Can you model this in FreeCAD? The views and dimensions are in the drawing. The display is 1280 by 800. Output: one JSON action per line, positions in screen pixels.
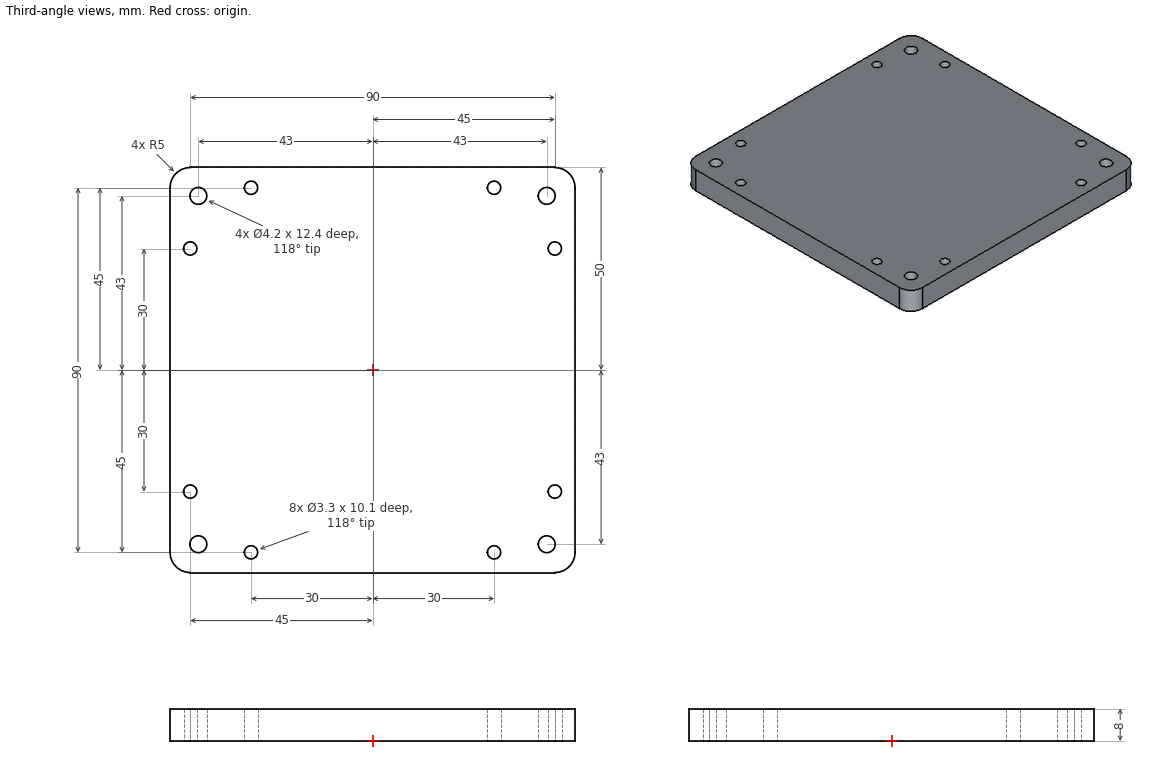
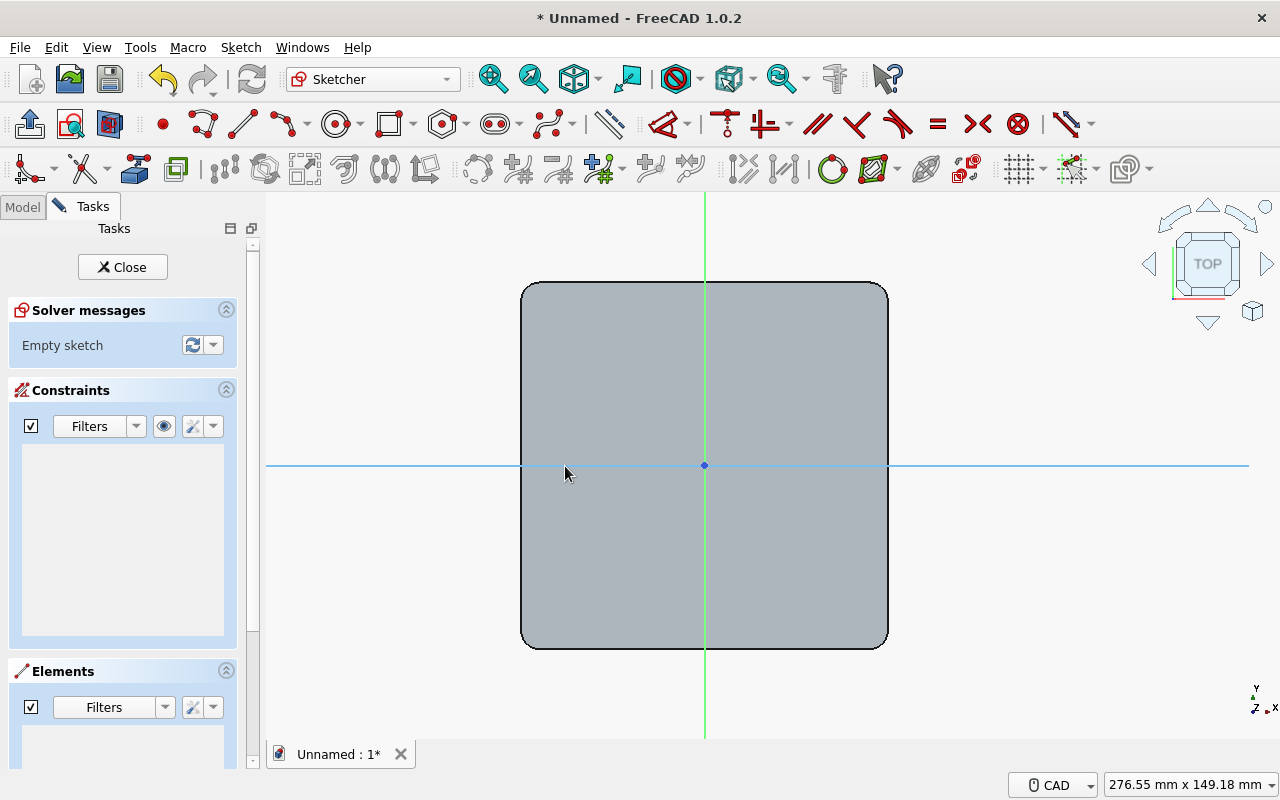
{"action": "key", "text": "g c"}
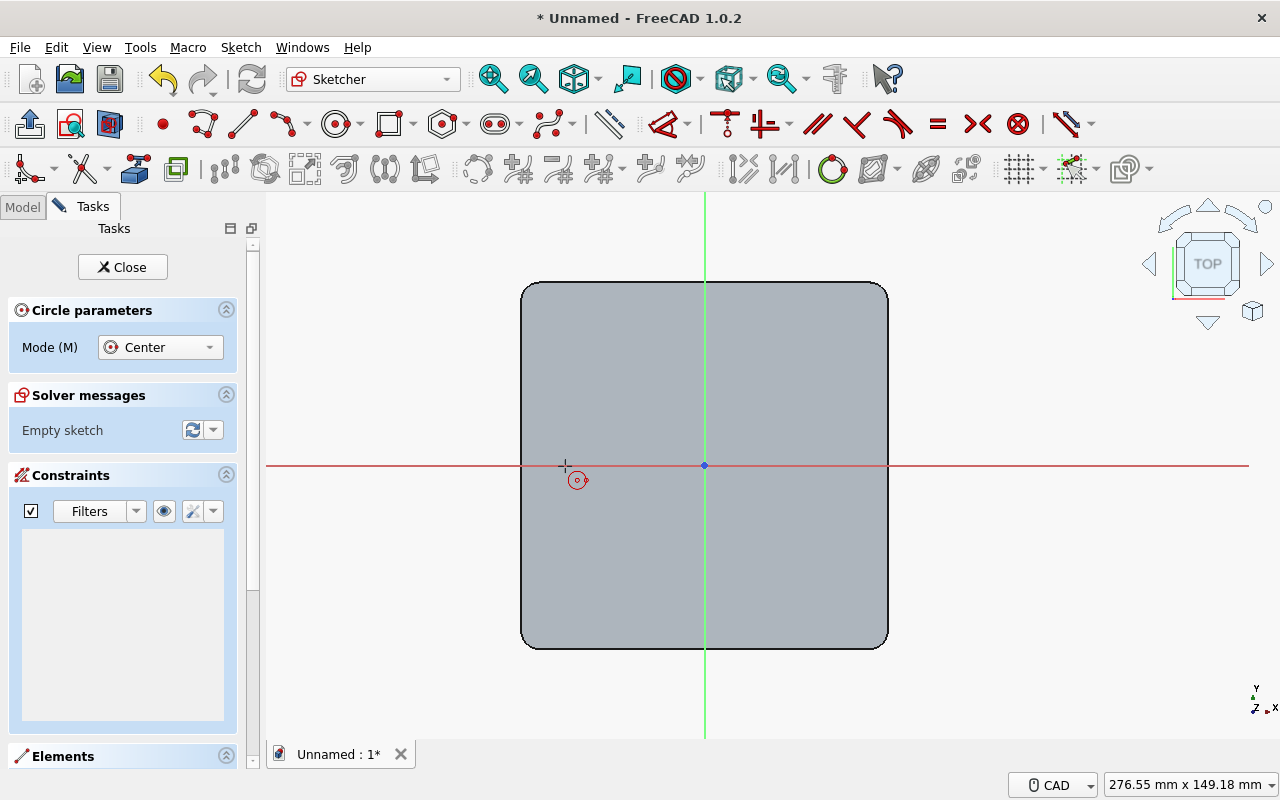
{"action": "scroll", "coordinate": [547, 308], "scroll_direction": "up", "scroll_amount": 6}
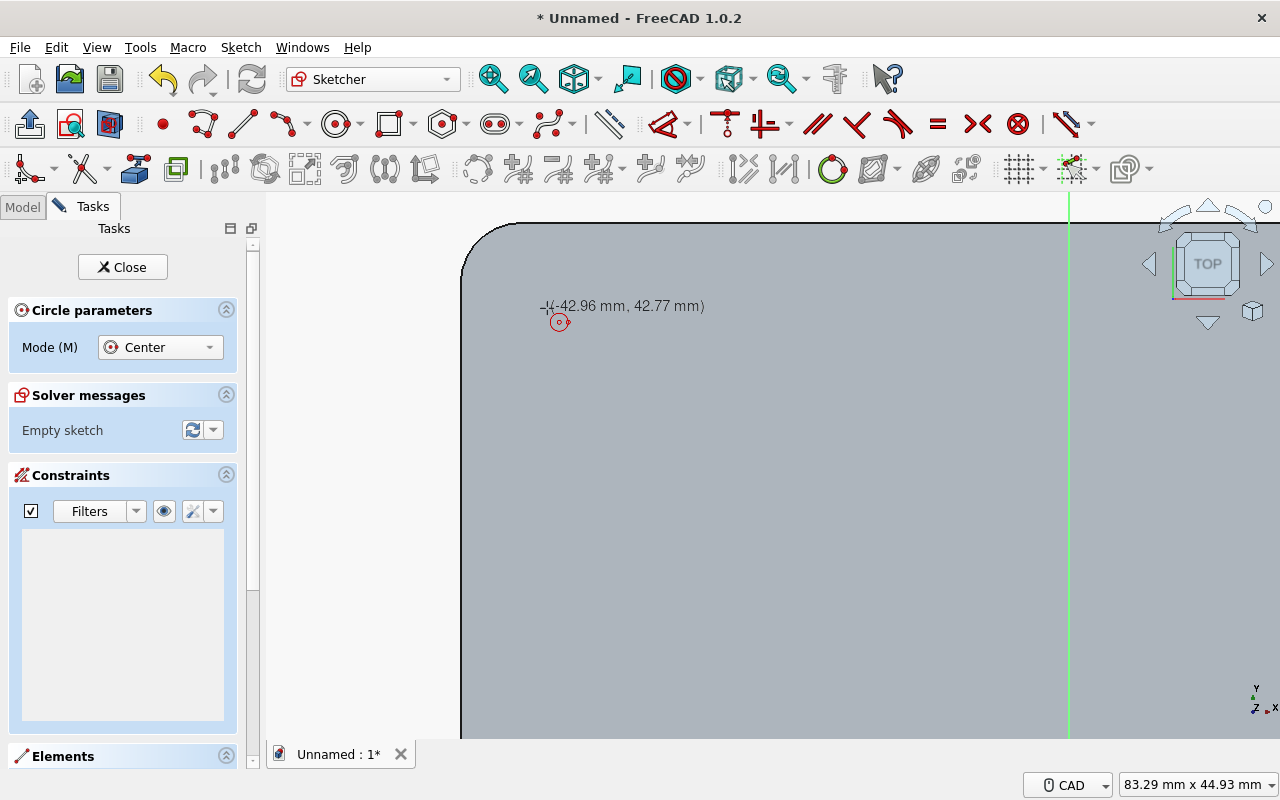
{"action": "left_click", "coordinate": [546, 308]}
{"action": "mouse_move", "coordinate": [564, 290]}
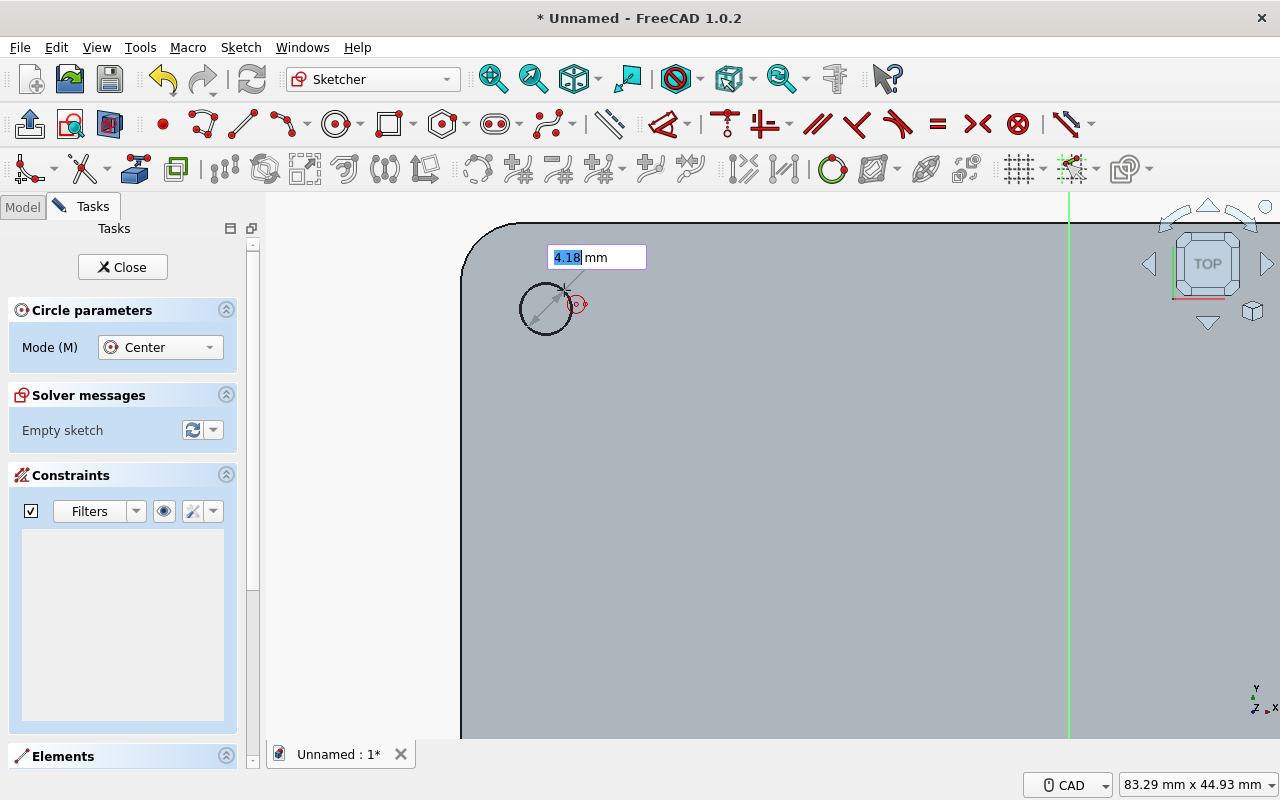
{"action": "type", "text": "4.2"}
{"action": "key", "text": "Return"}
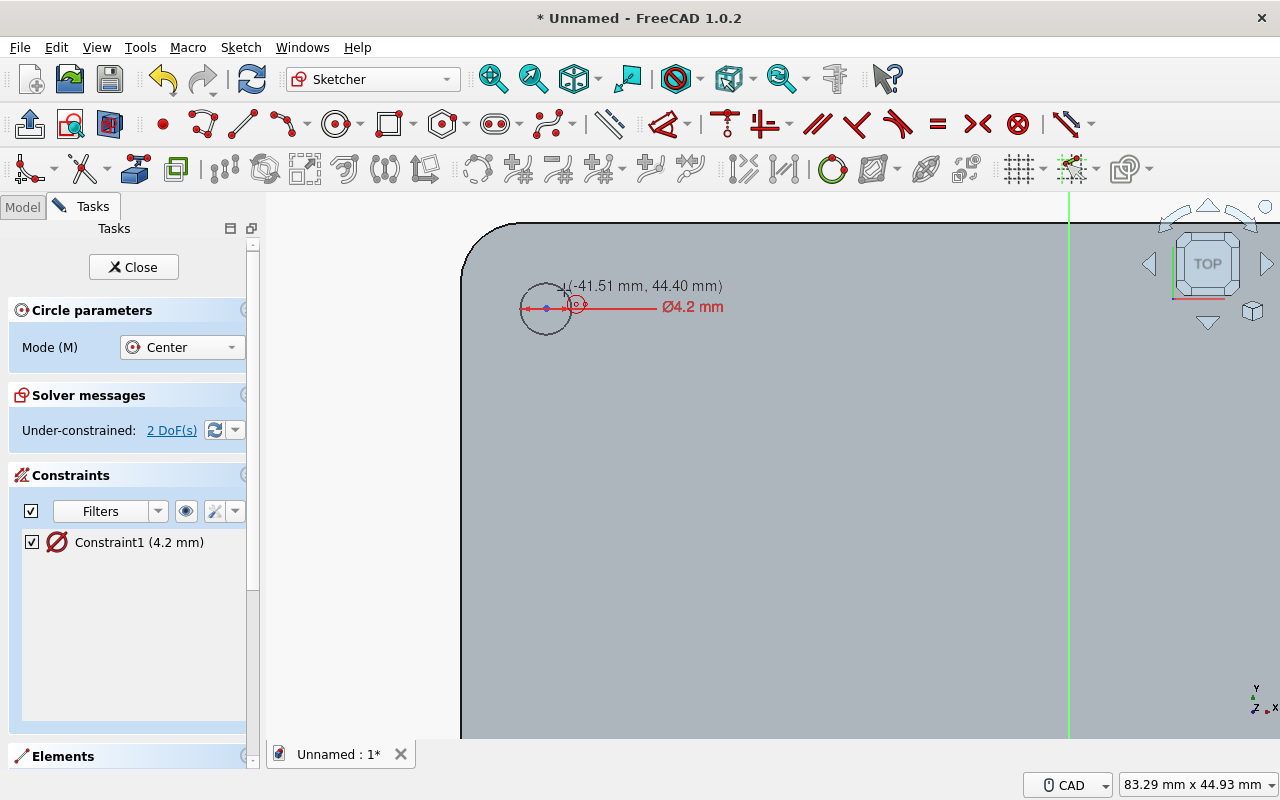
{"action": "scroll", "coordinate": [547, 308], "scroll_direction": "down", "scroll_amount": 6}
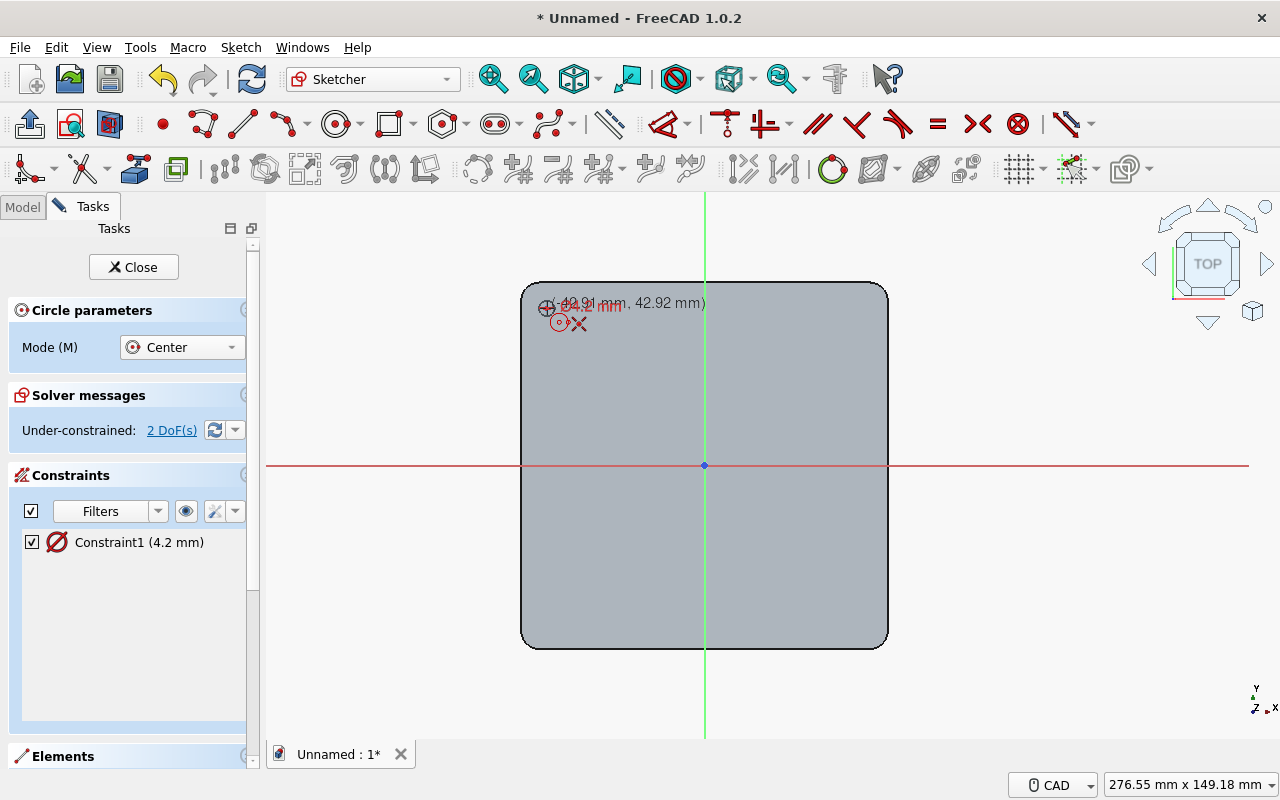
{"action": "scroll", "coordinate": [862, 308], "scroll_direction": "up", "scroll_amount": 6}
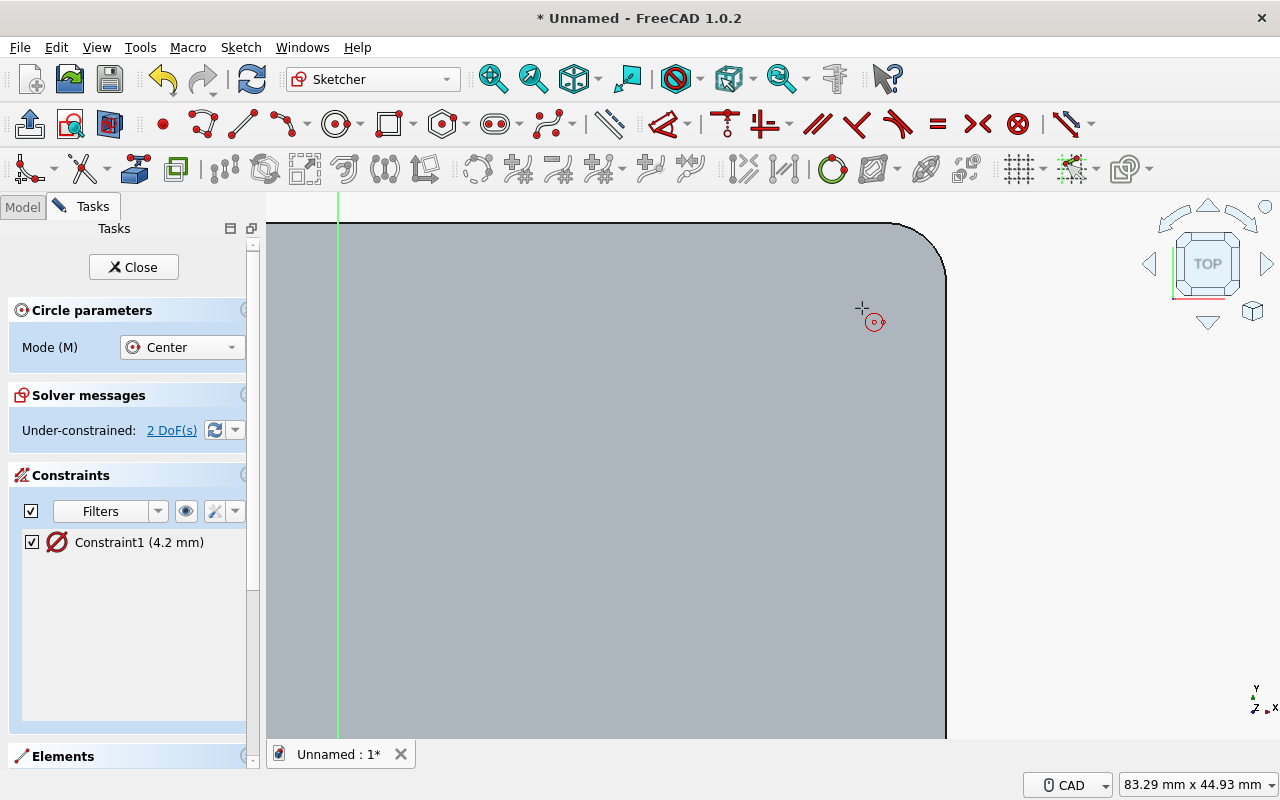
{"action": "left_click", "coordinate": [861, 308]}
{"action": "mouse_move", "coordinate": [879, 290]}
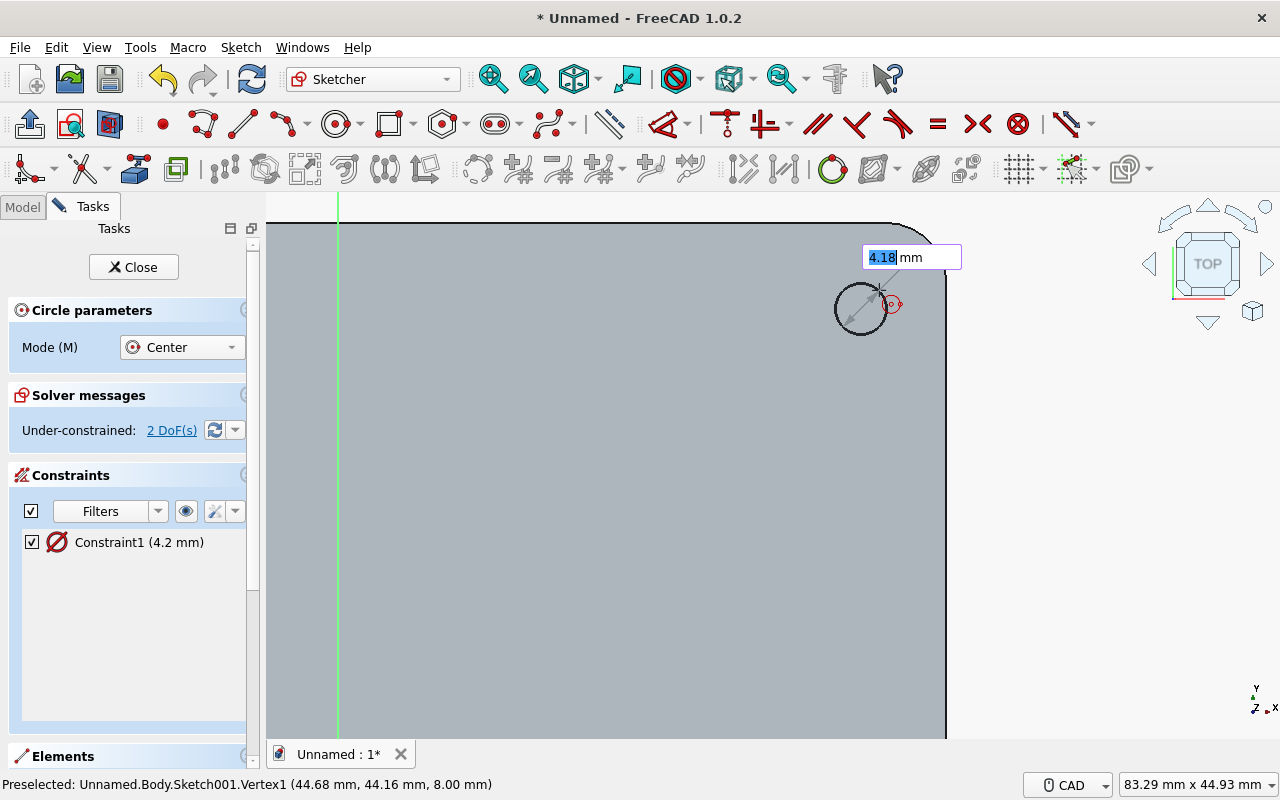
{"action": "type", "text": "4.2"}
{"action": "key", "text": "Return"}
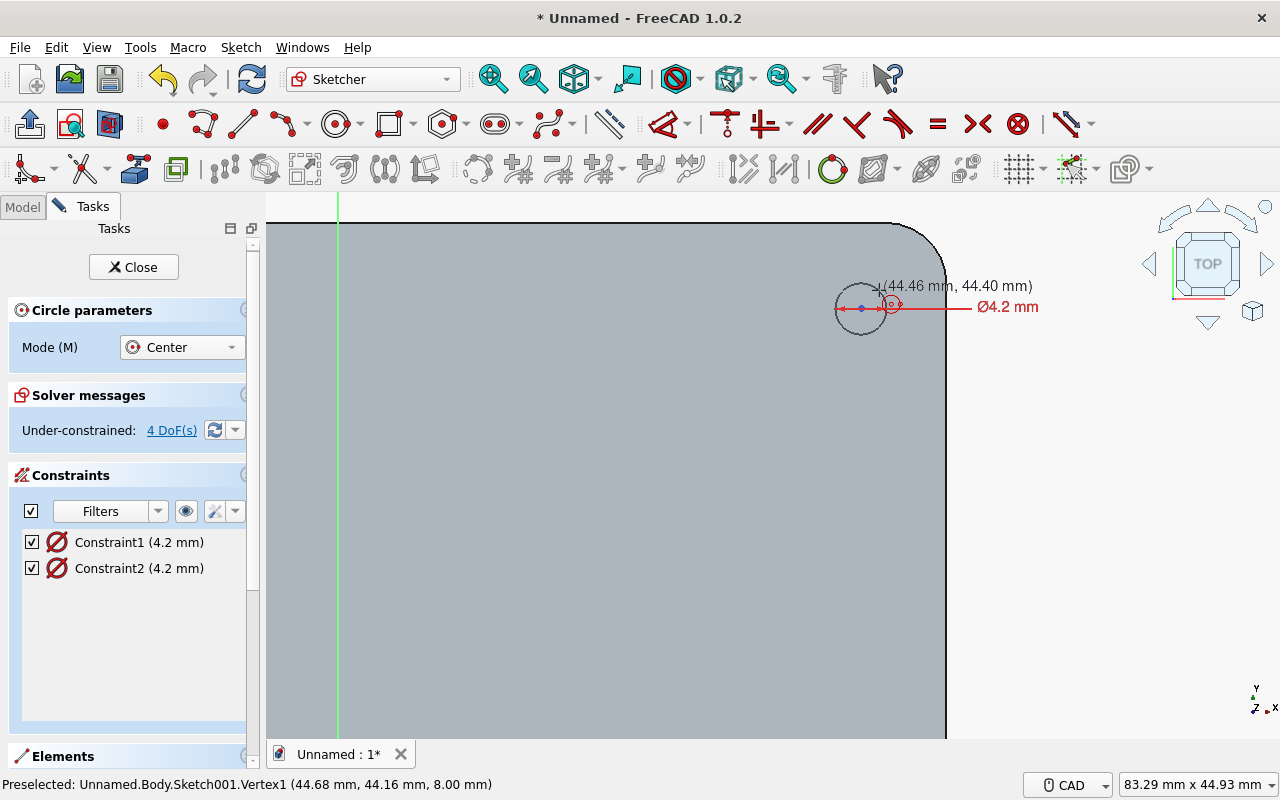
{"action": "scroll", "coordinate": [863, 308], "scroll_direction": "down", "scroll_amount": 6}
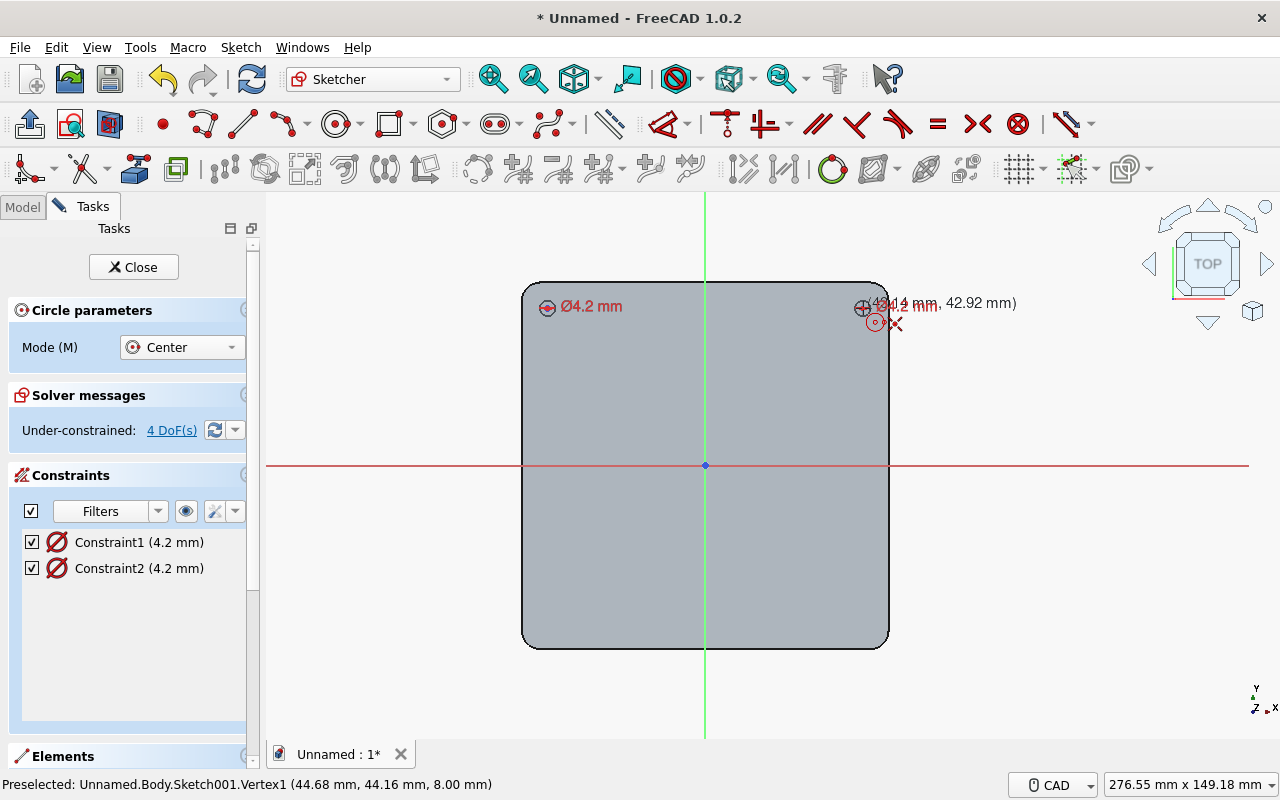
{"action": "scroll", "coordinate": [863, 623], "scroll_direction": "up", "scroll_amount": 6}